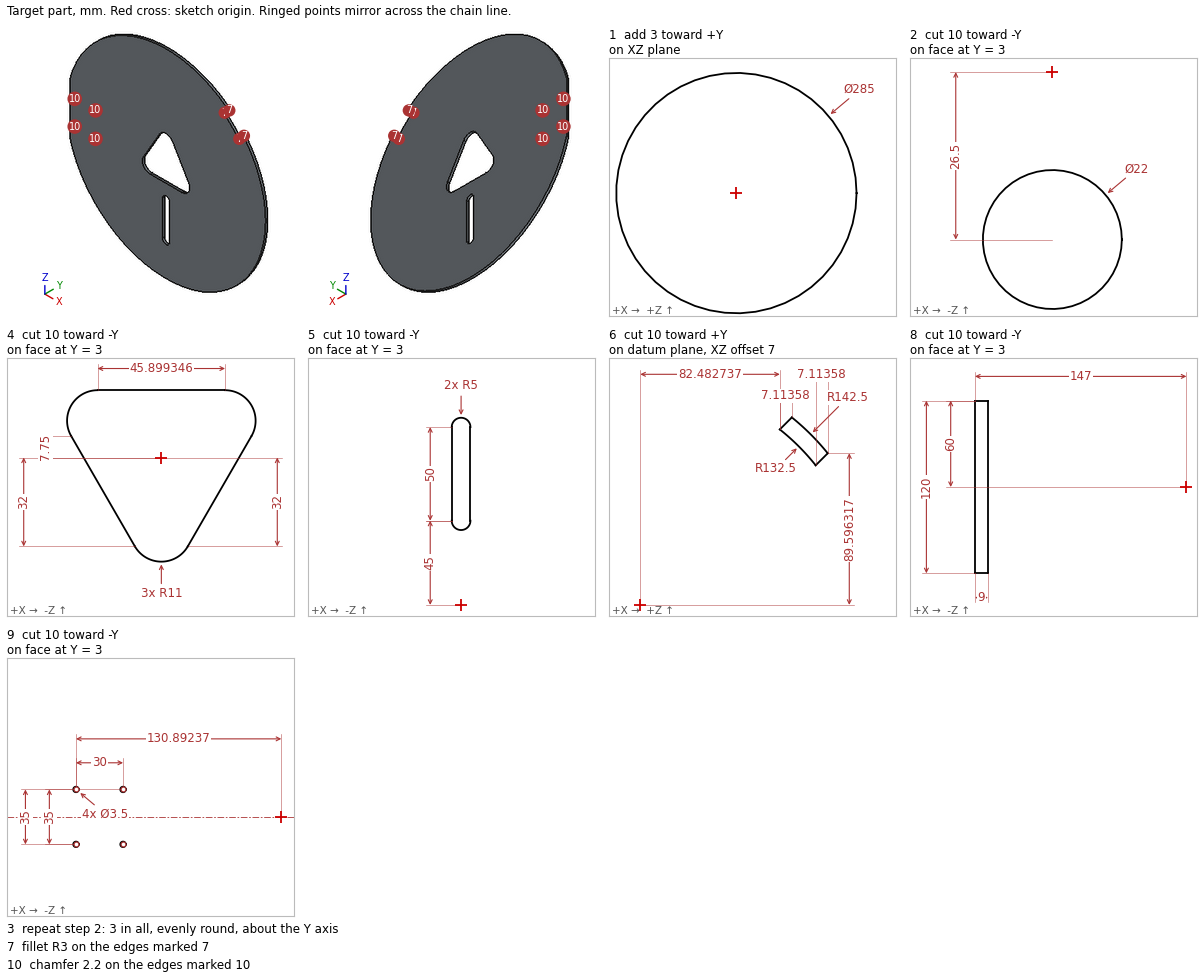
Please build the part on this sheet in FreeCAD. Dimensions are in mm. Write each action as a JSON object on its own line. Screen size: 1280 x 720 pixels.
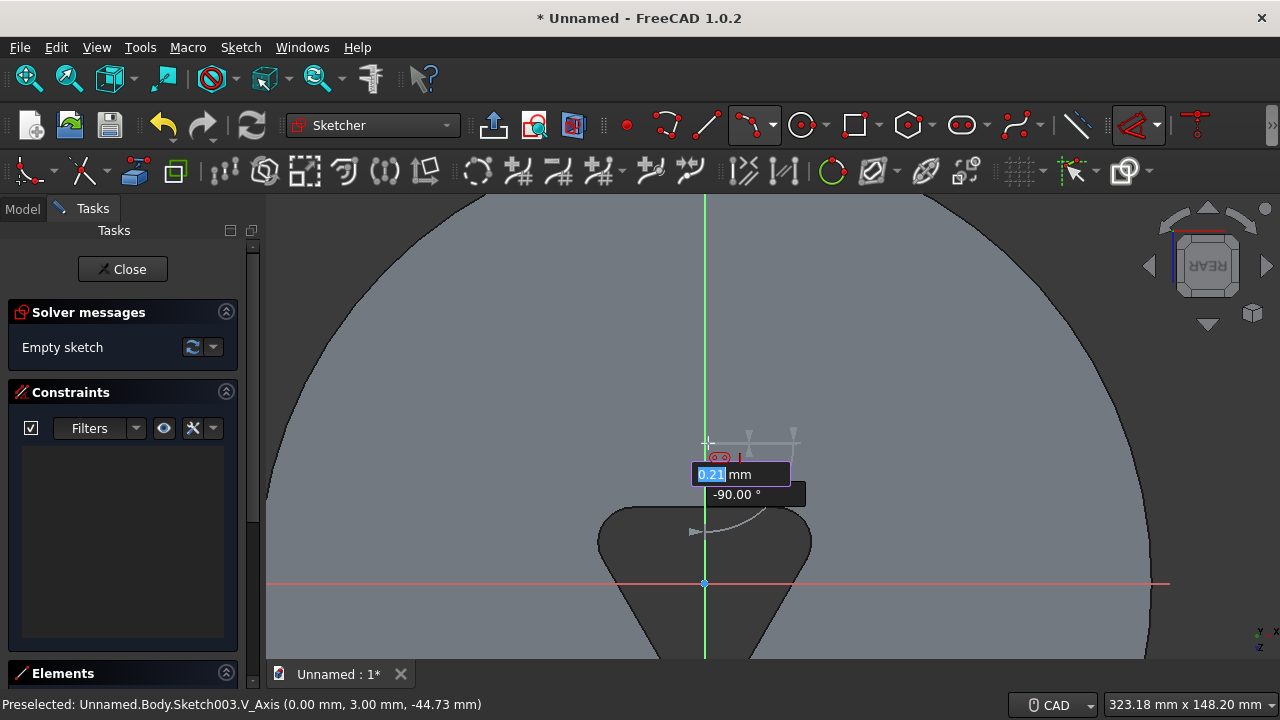
{"action": "left_click", "coordinate": [714, 285]}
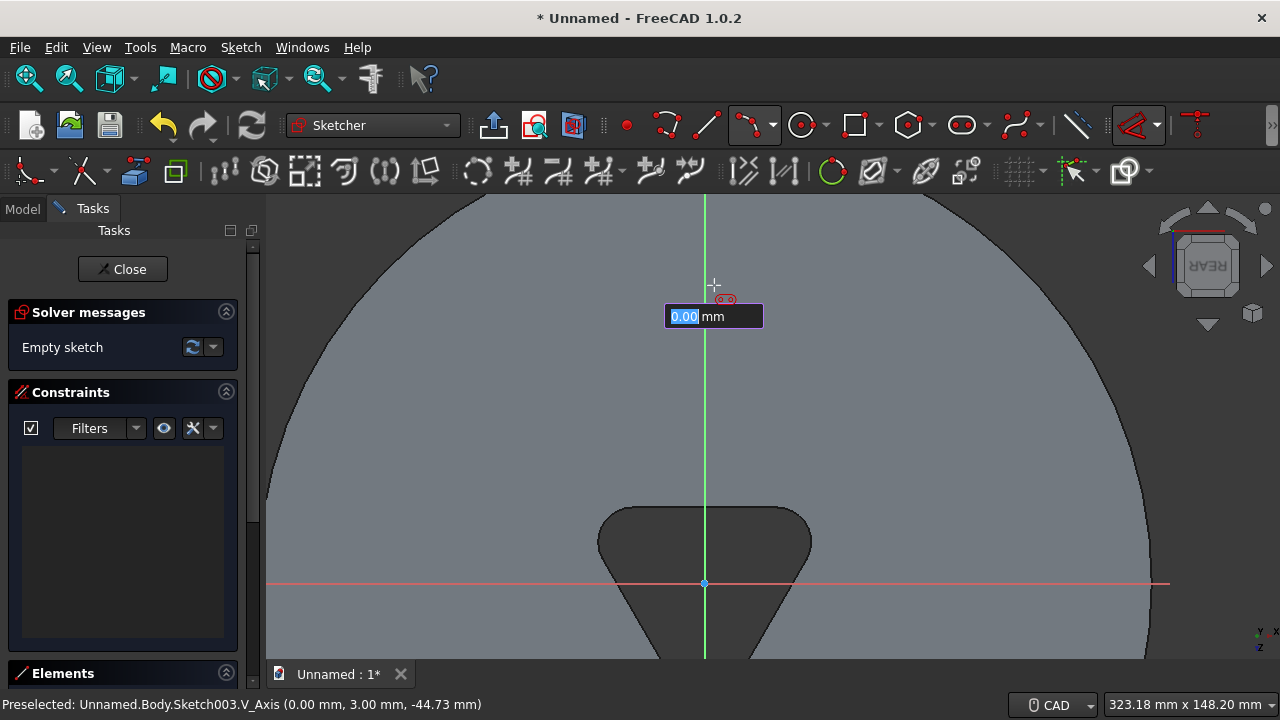
{"action": "left_click", "coordinate": [689, 364]}
{"action": "key", "text": "Escape"}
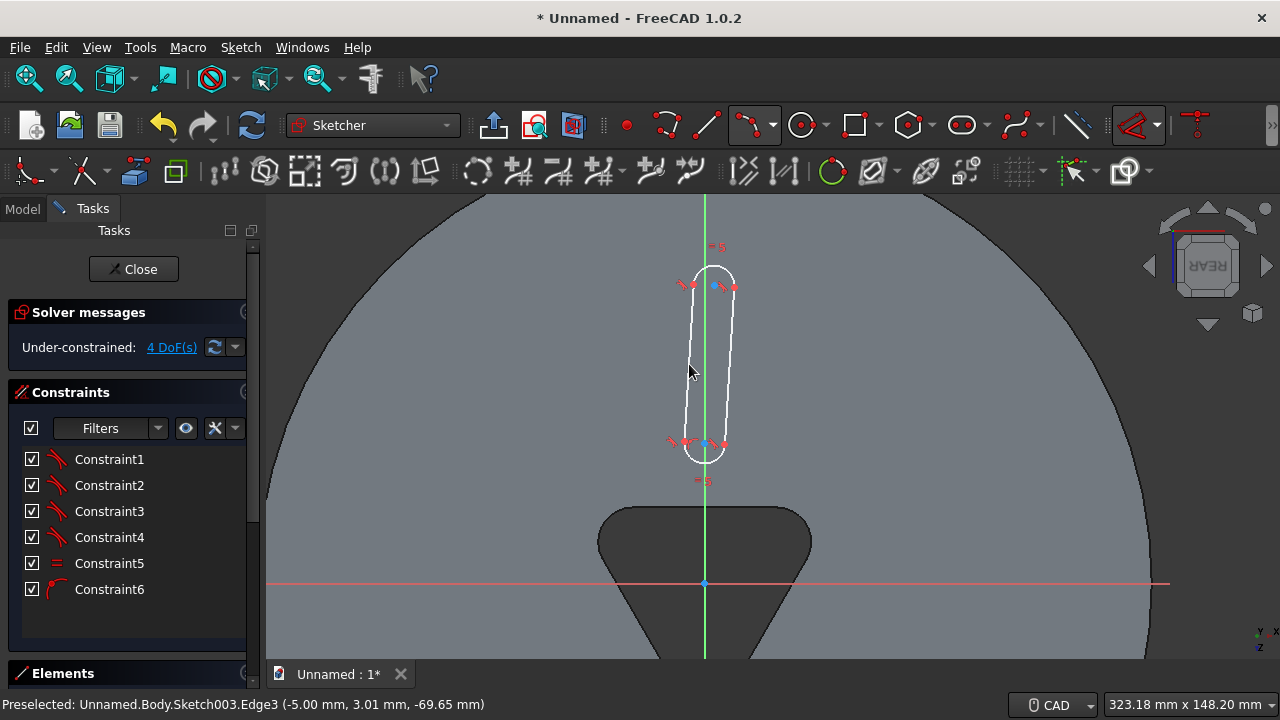
{"action": "left_click", "coordinate": [687, 395]}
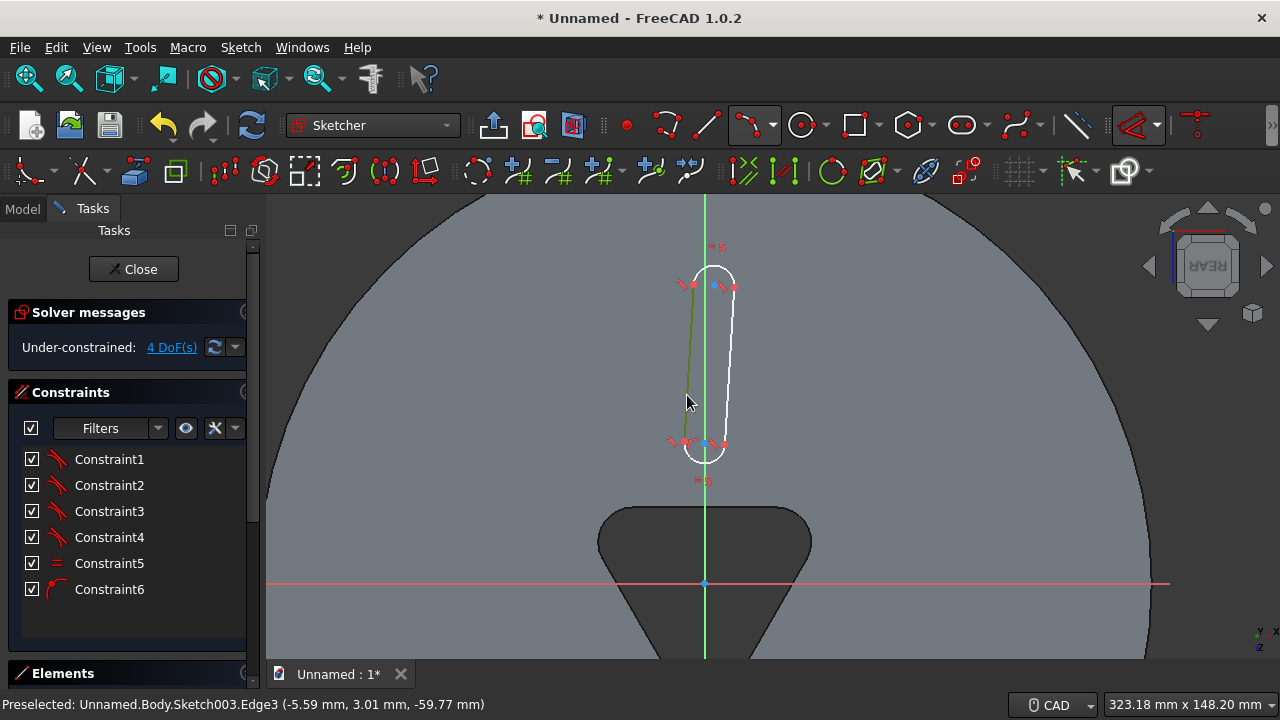
{"action": "key", "text": "v"}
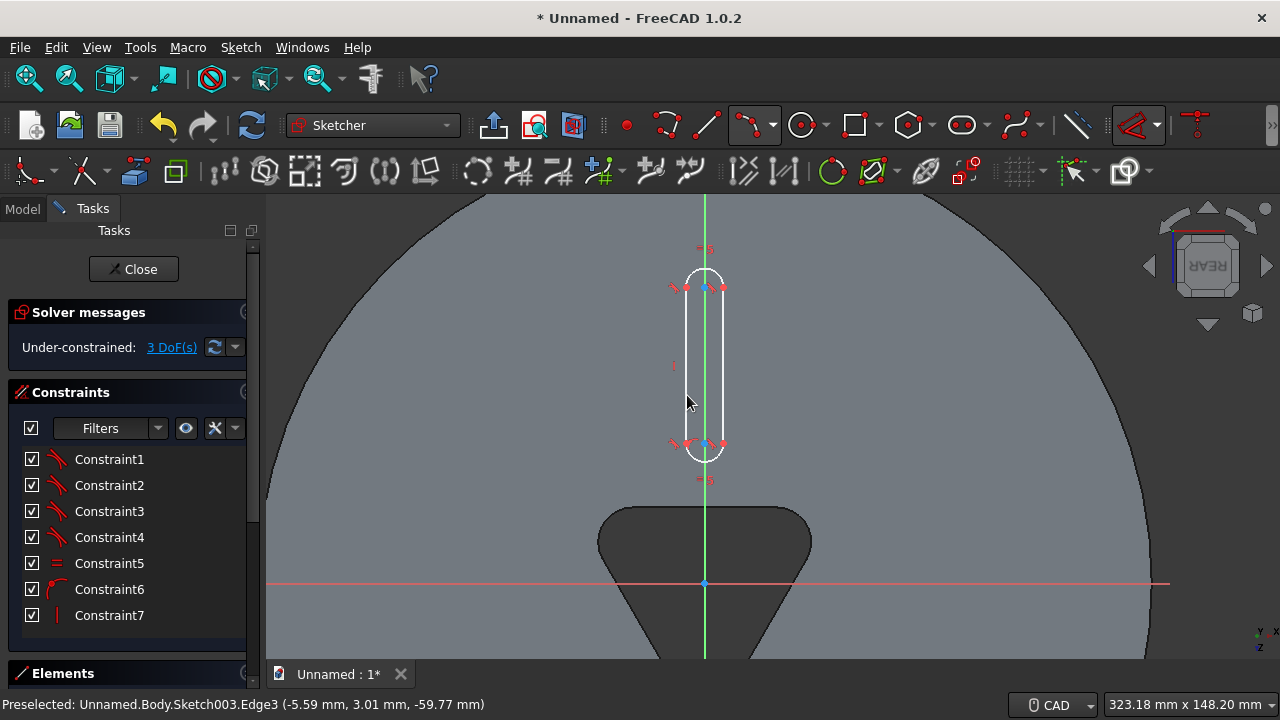
{"action": "scroll", "coordinate": [694, 458], "scroll_direction": "up", "scroll_amount": 5}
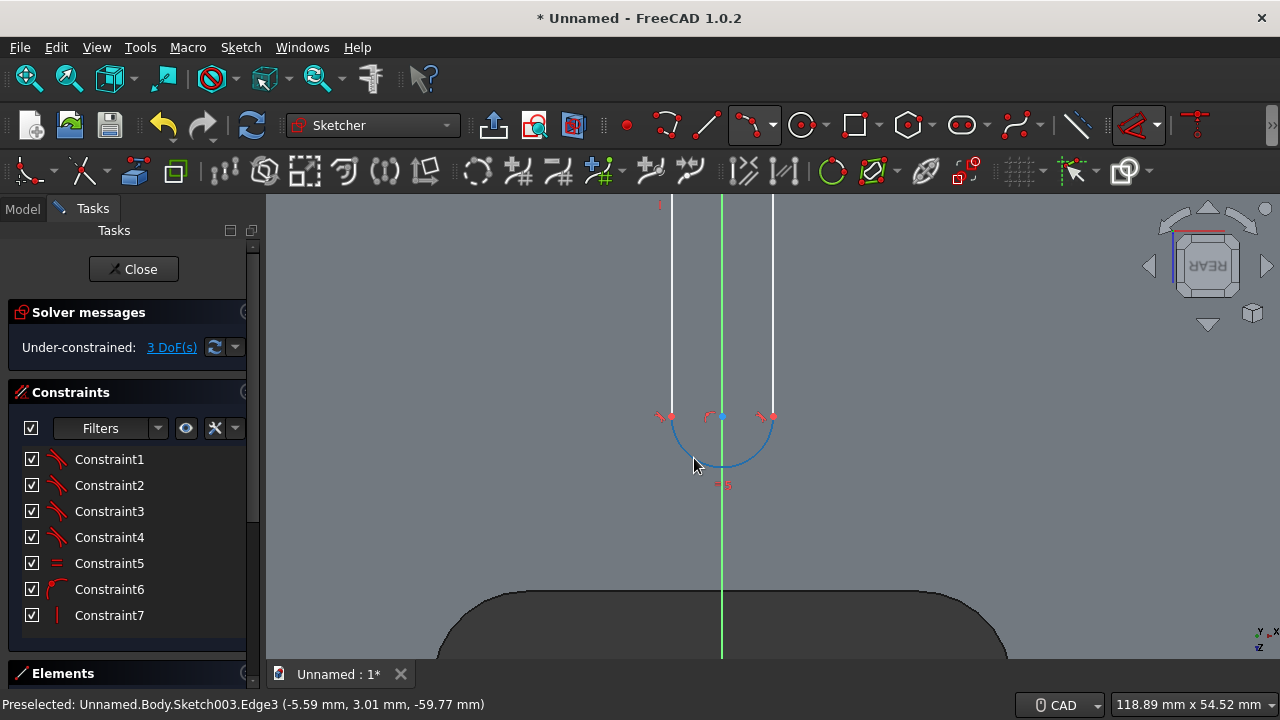
{"action": "left_click", "coordinate": [693, 458]}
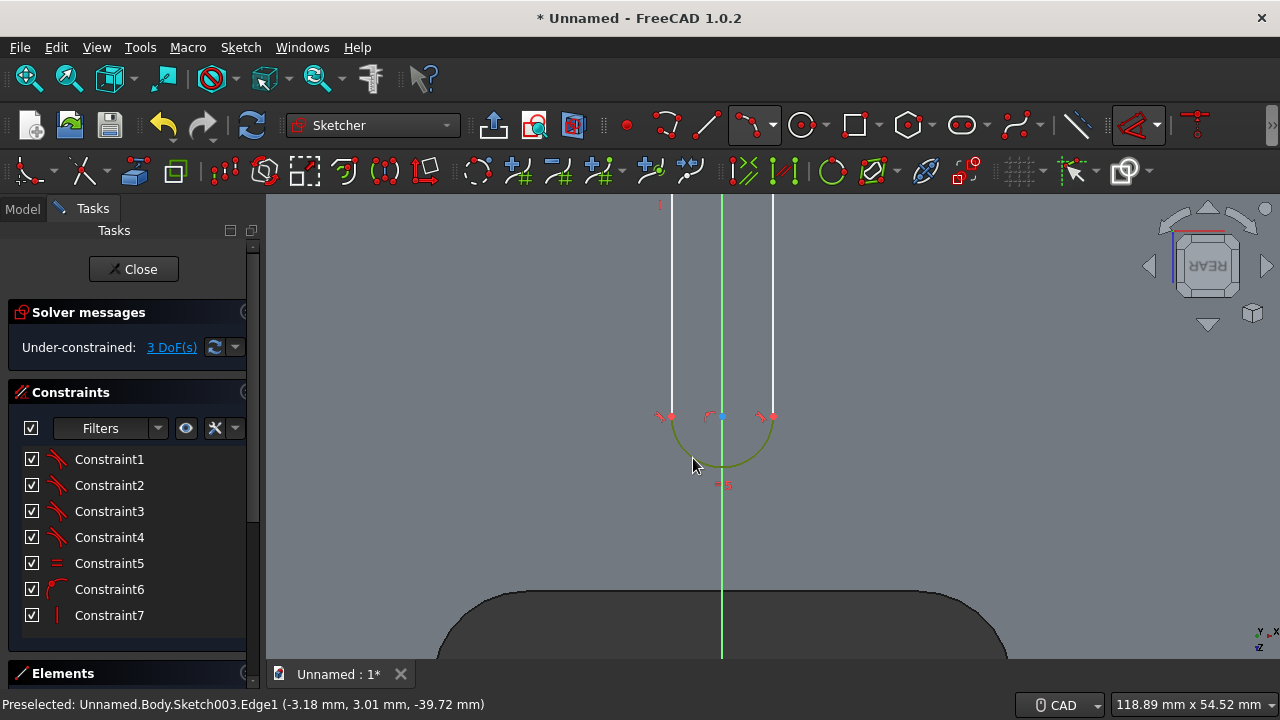
{"action": "left_click", "coordinate": [1160, 126]}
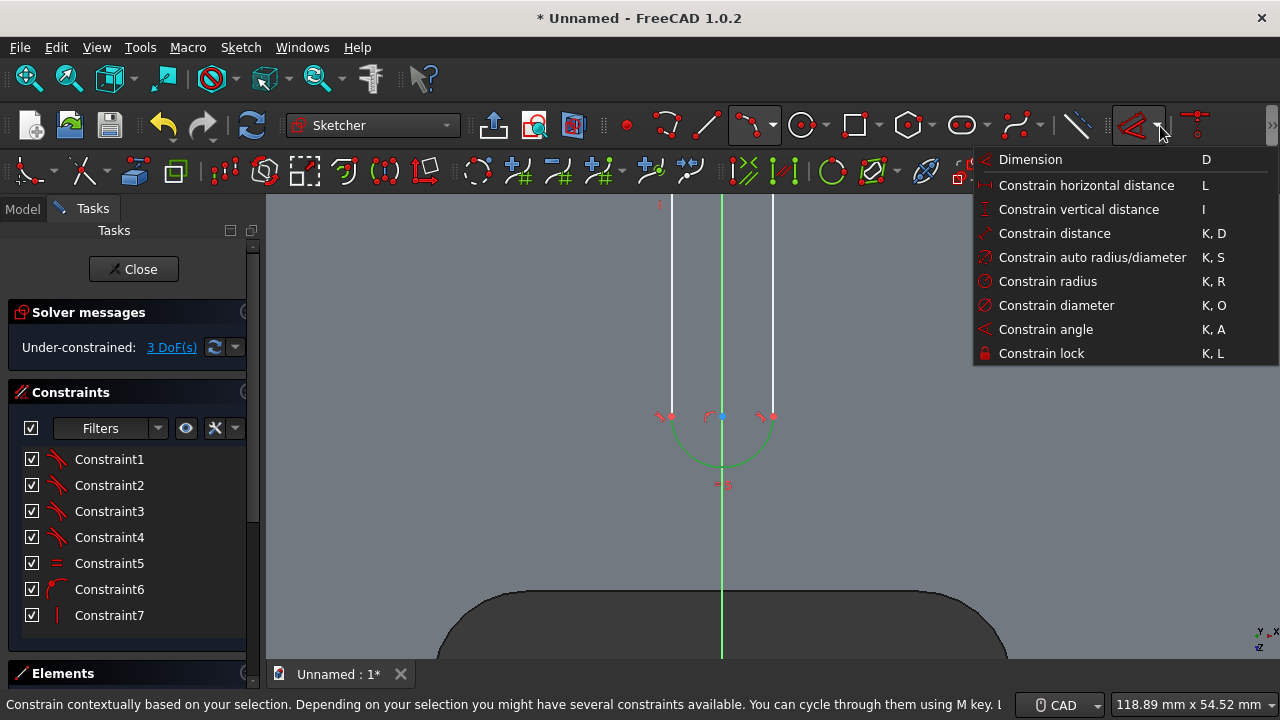
{"action": "left_click", "coordinate": [1126, 281]}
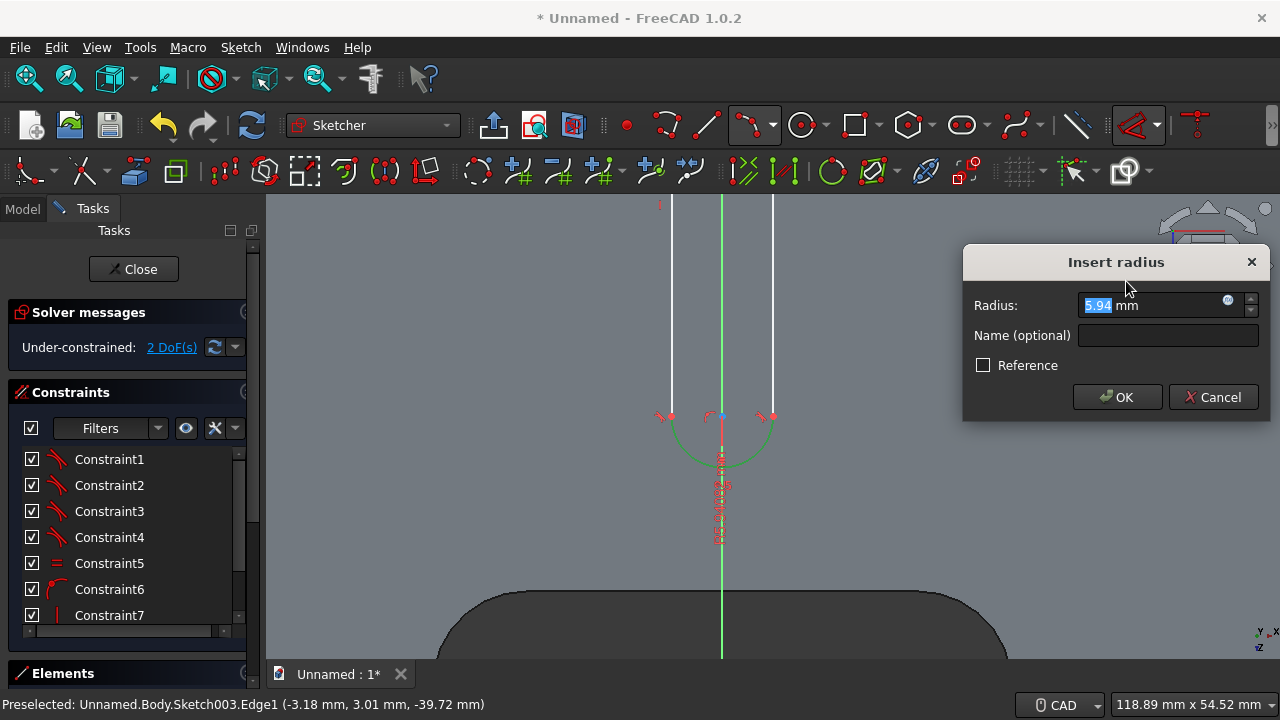
{"action": "type", "text": "5"}
{"action": "key", "text": "Return"}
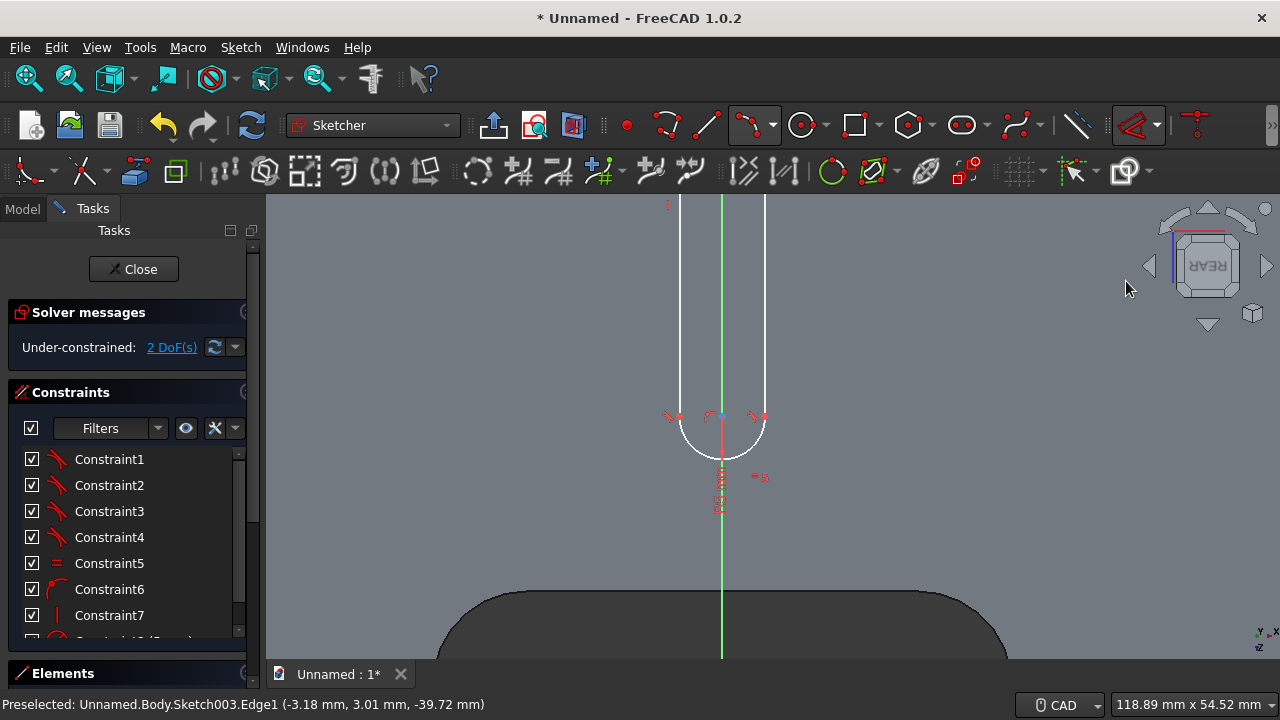
{"action": "left_click", "coordinate": [680, 290]}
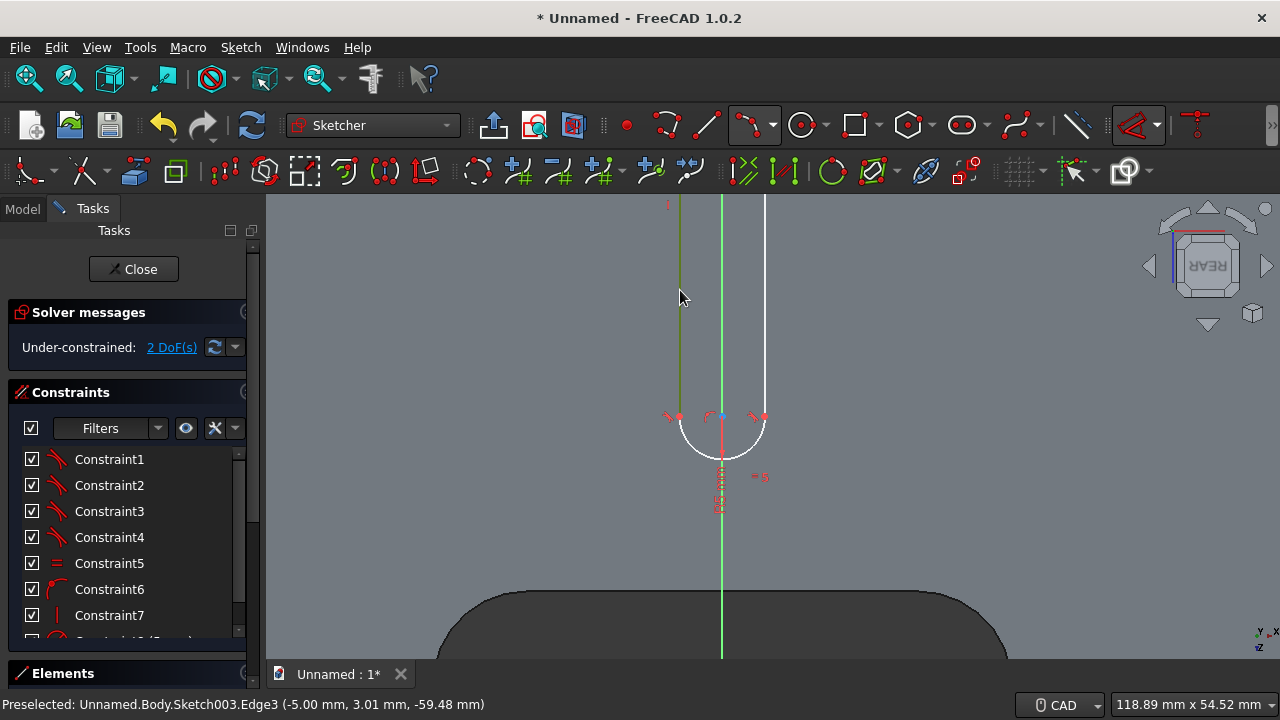
{"action": "left_click", "coordinate": [1160, 126]}